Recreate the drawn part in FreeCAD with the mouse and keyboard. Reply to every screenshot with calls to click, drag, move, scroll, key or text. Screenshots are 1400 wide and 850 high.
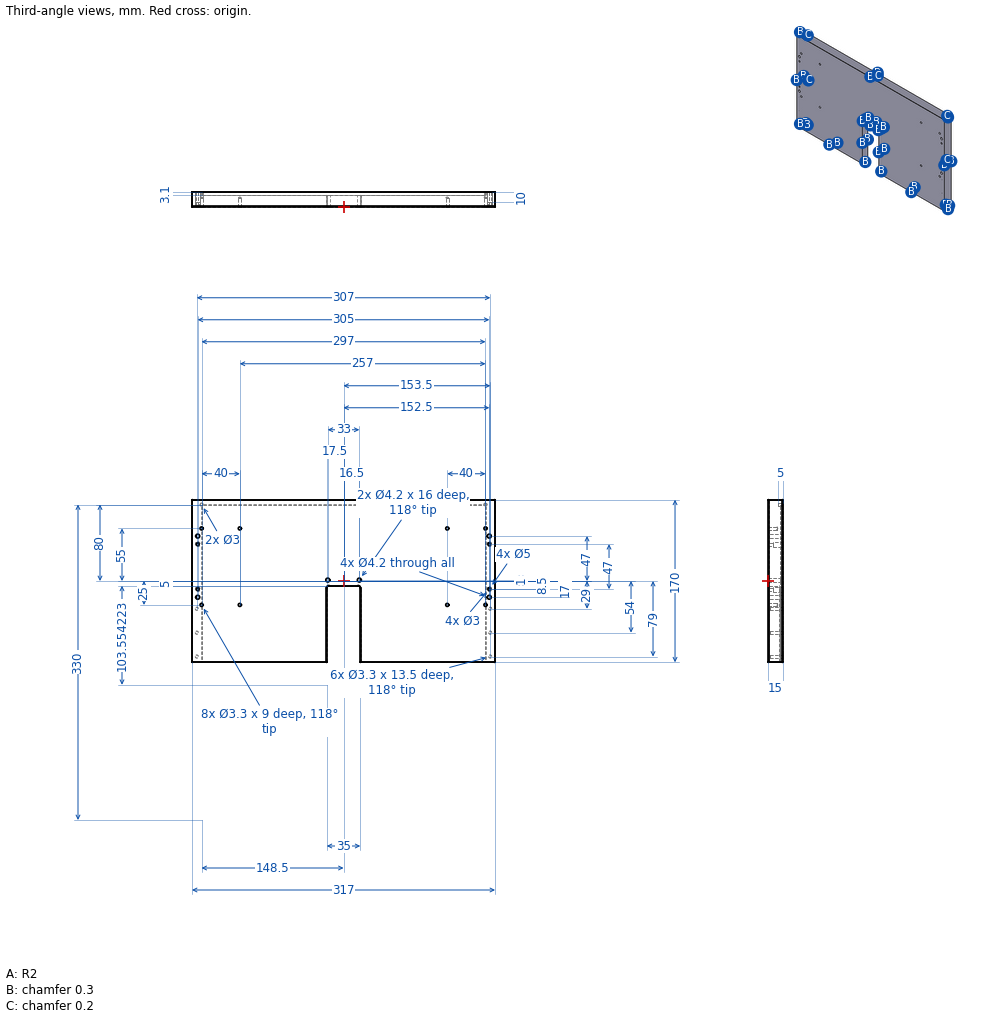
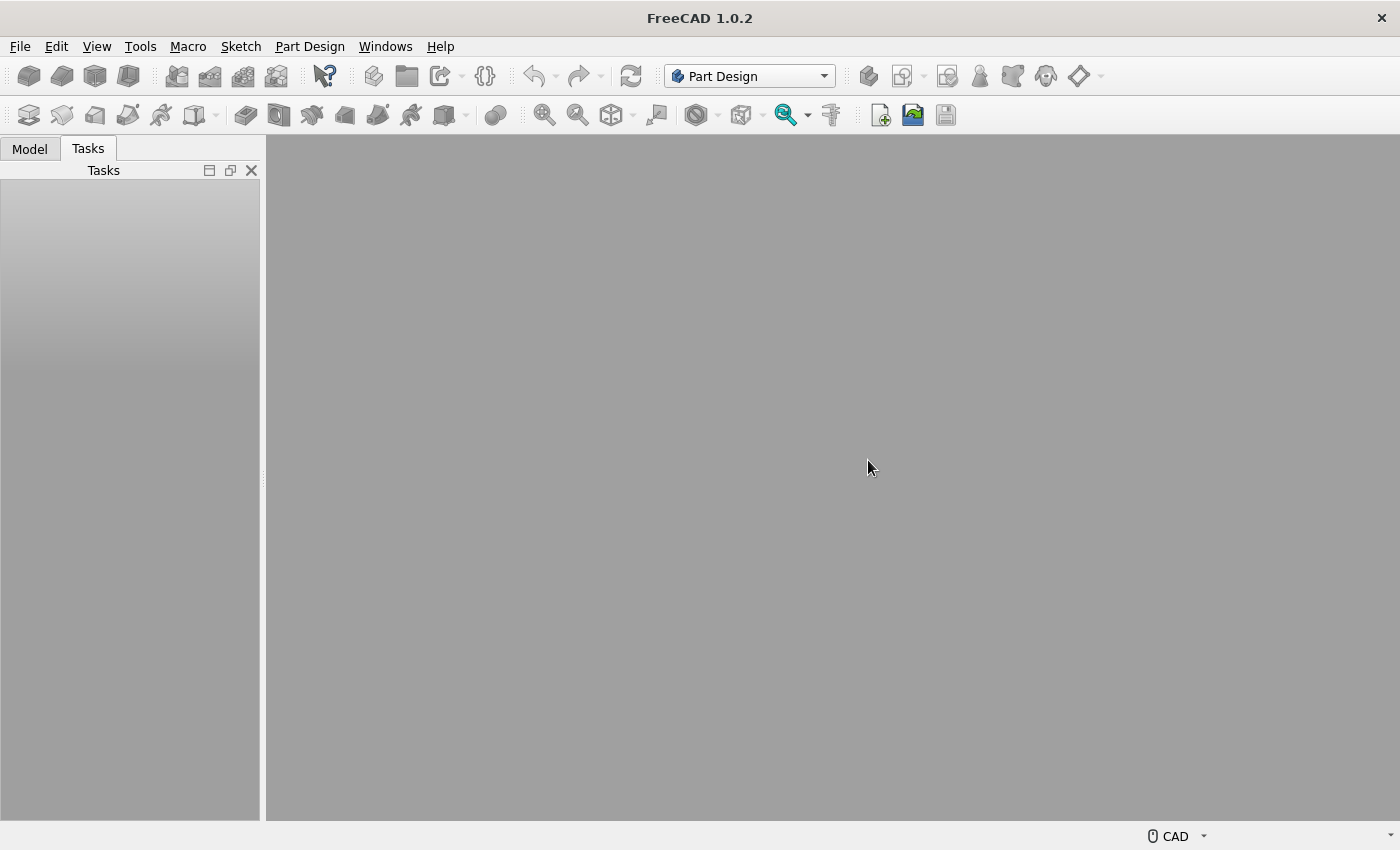
key(ctrl+n)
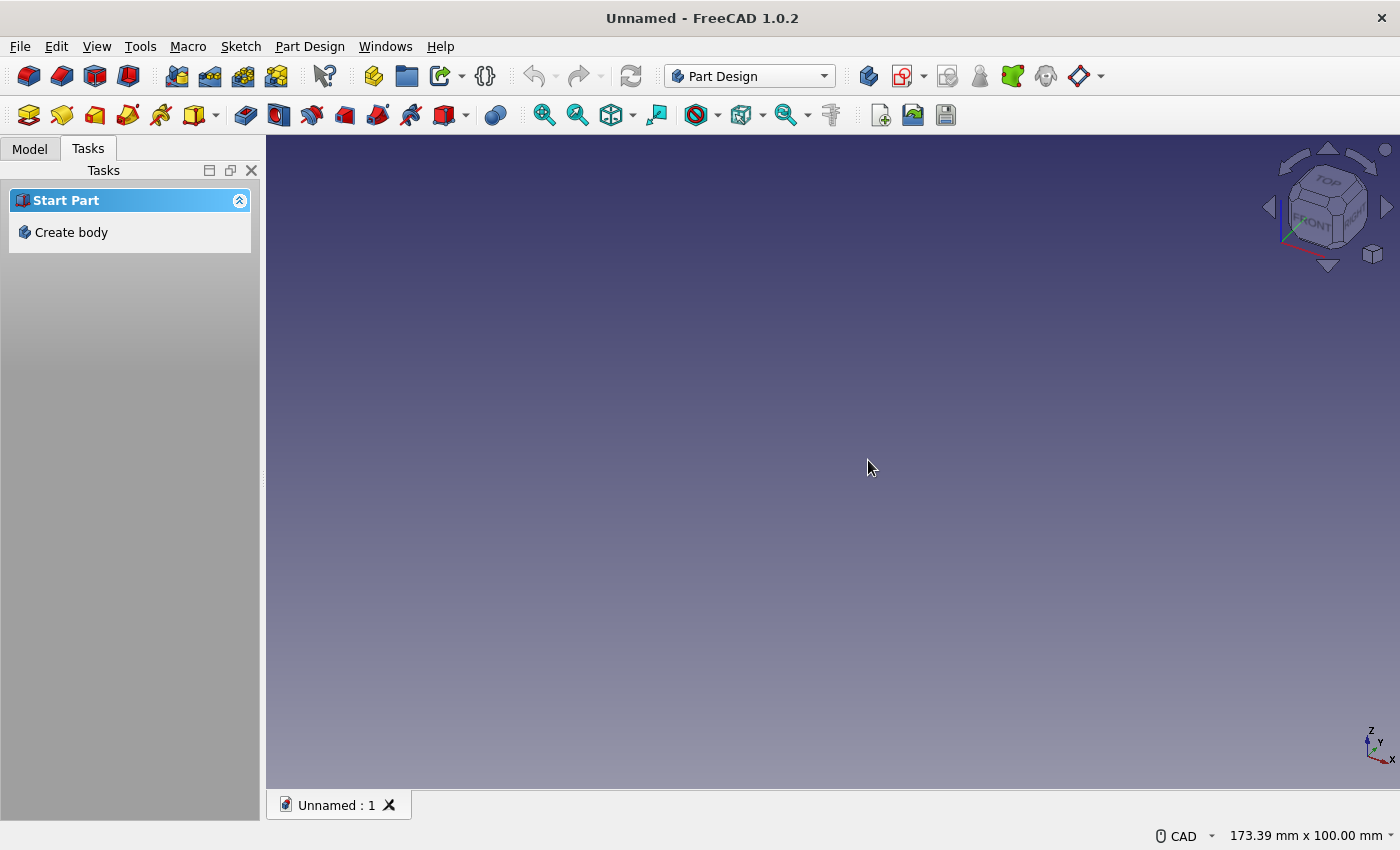
click(902, 76)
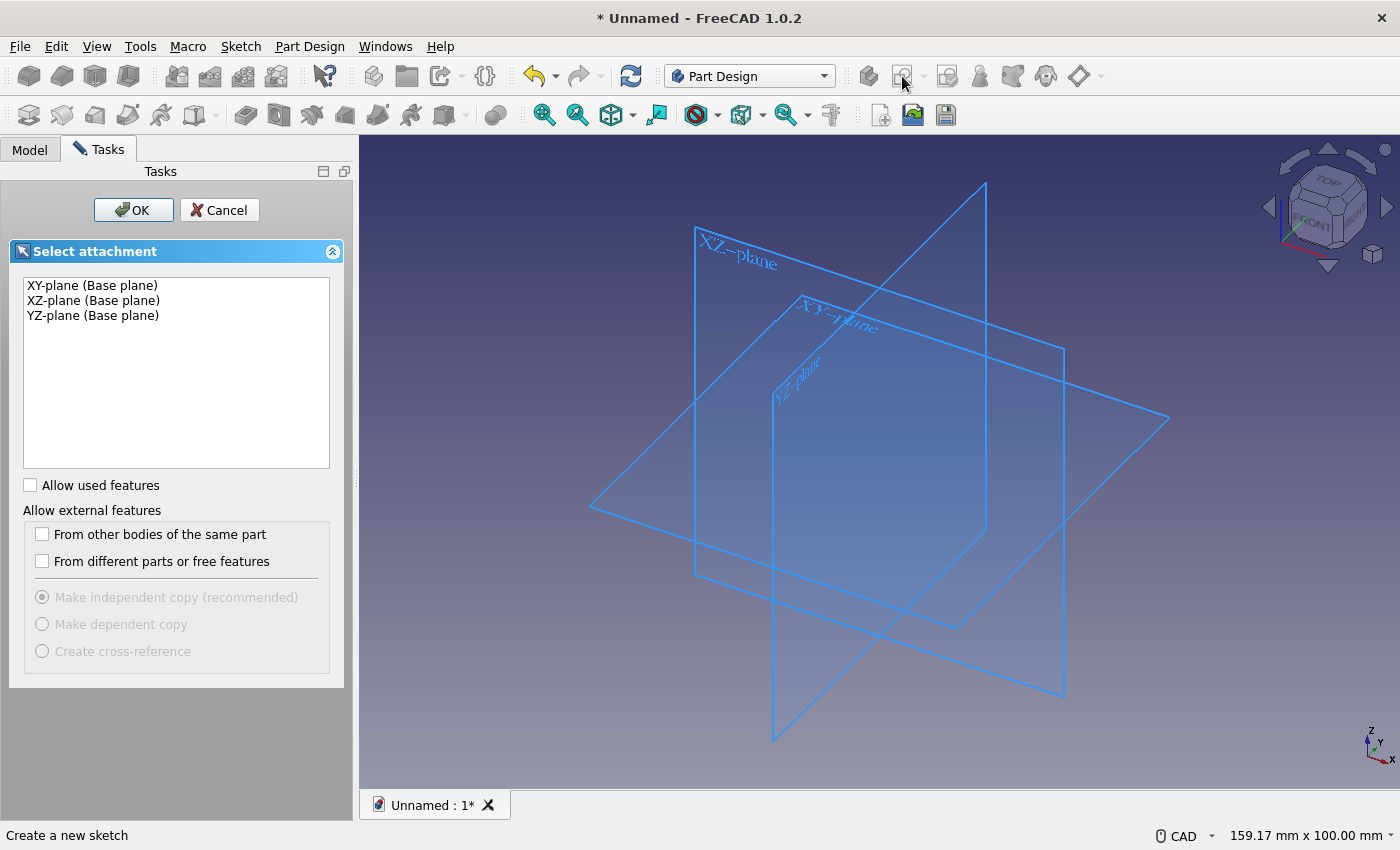
click(84, 300)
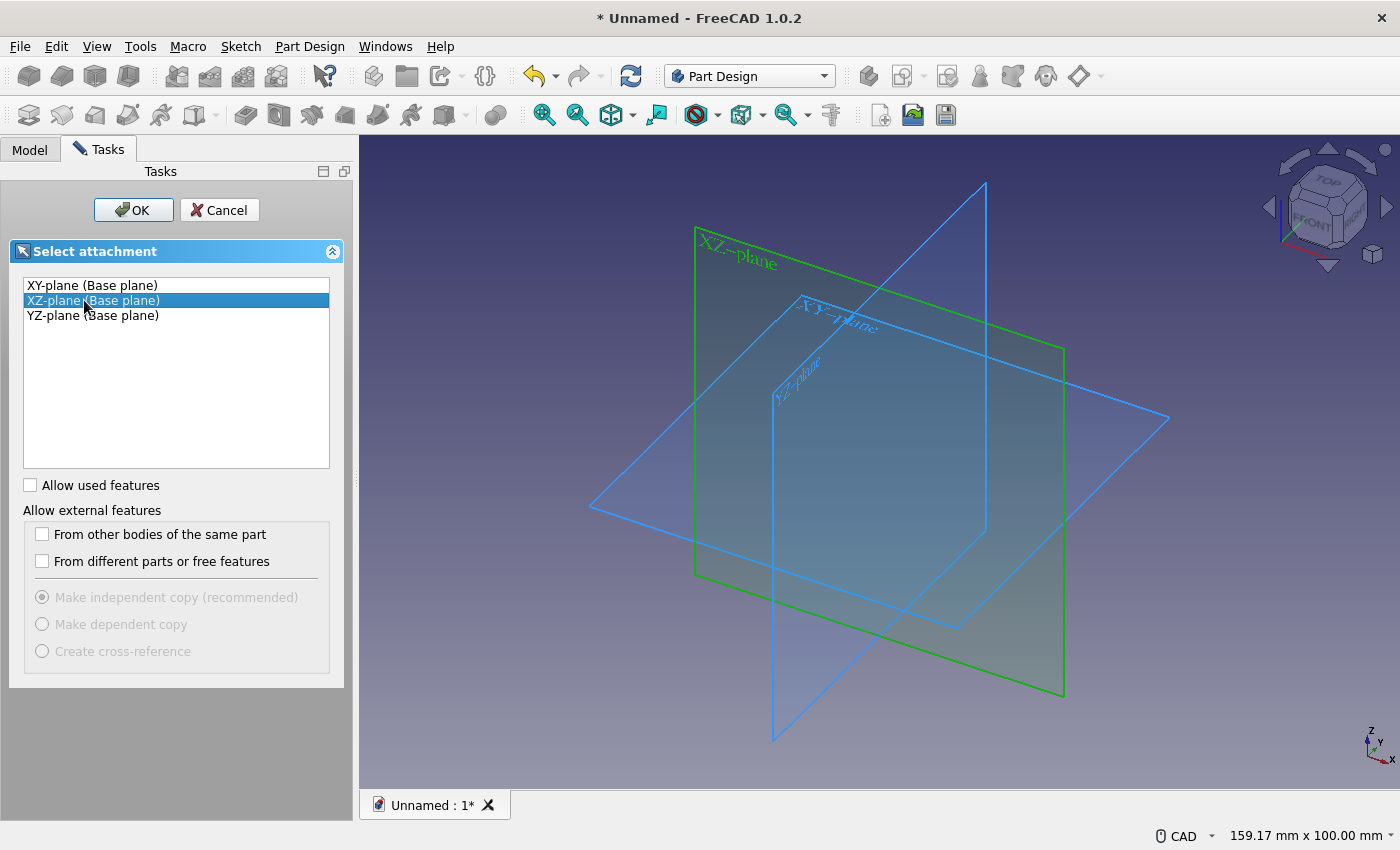
click(134, 210)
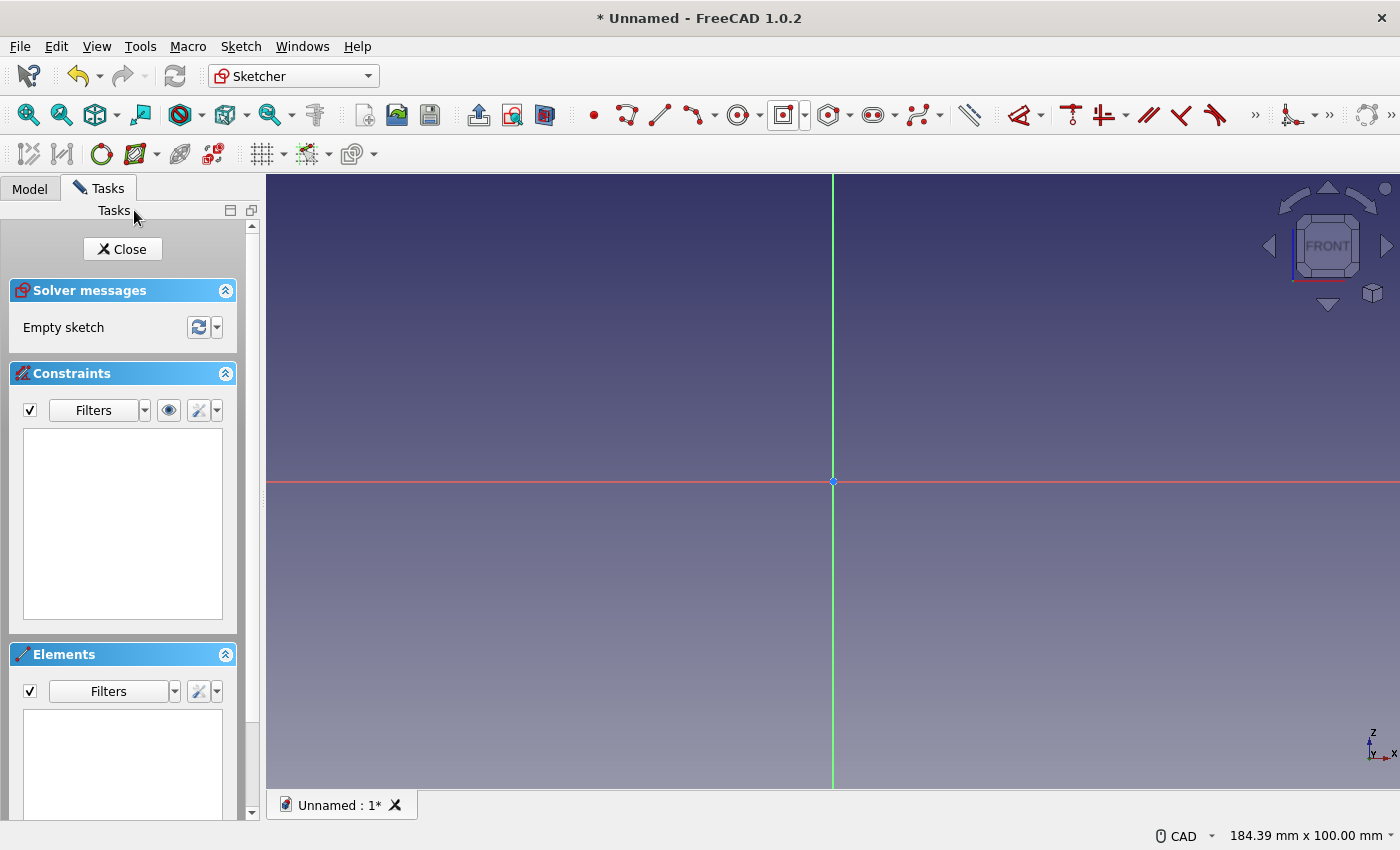
scroll(725, 482, down, 5)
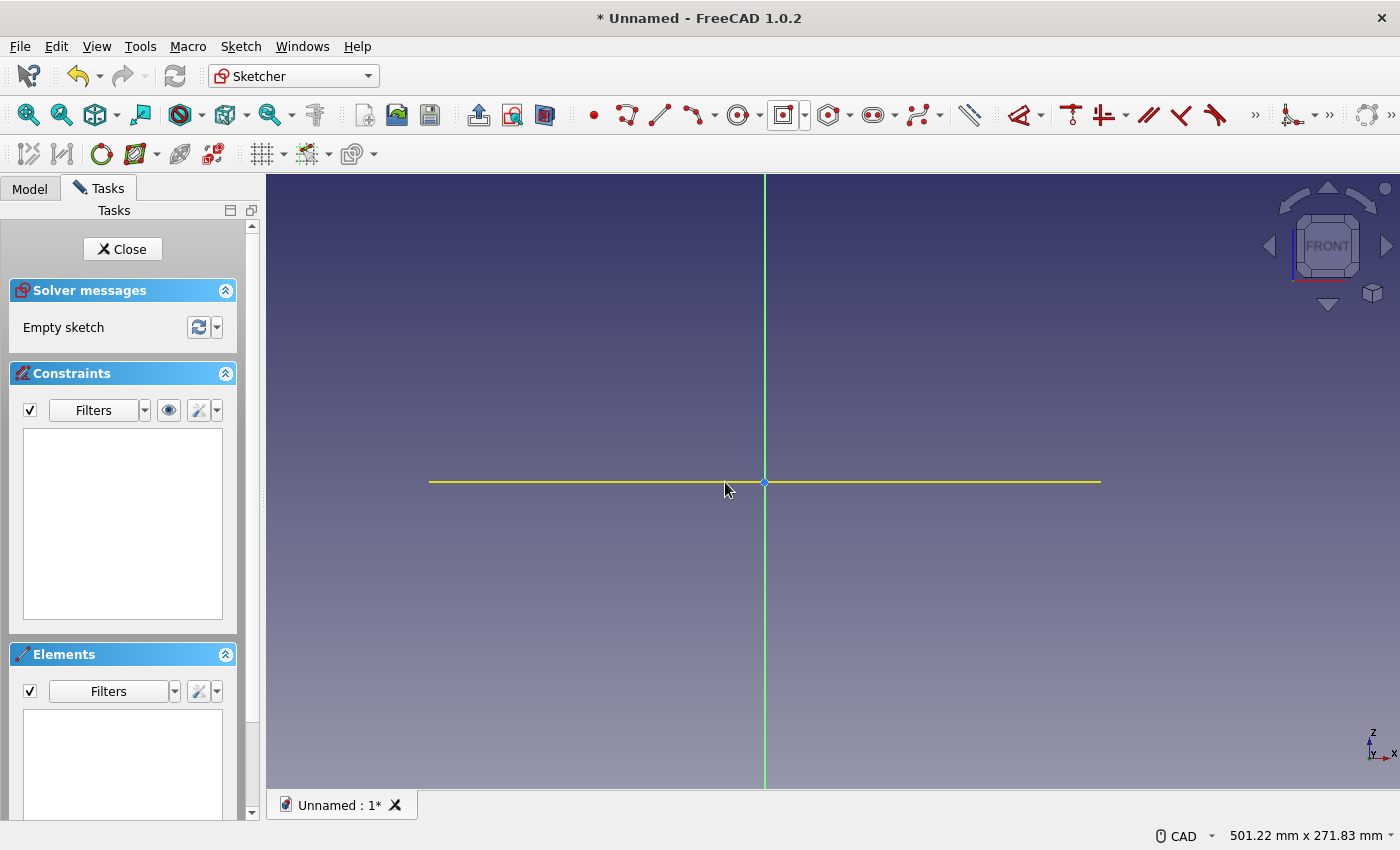
click(782, 116)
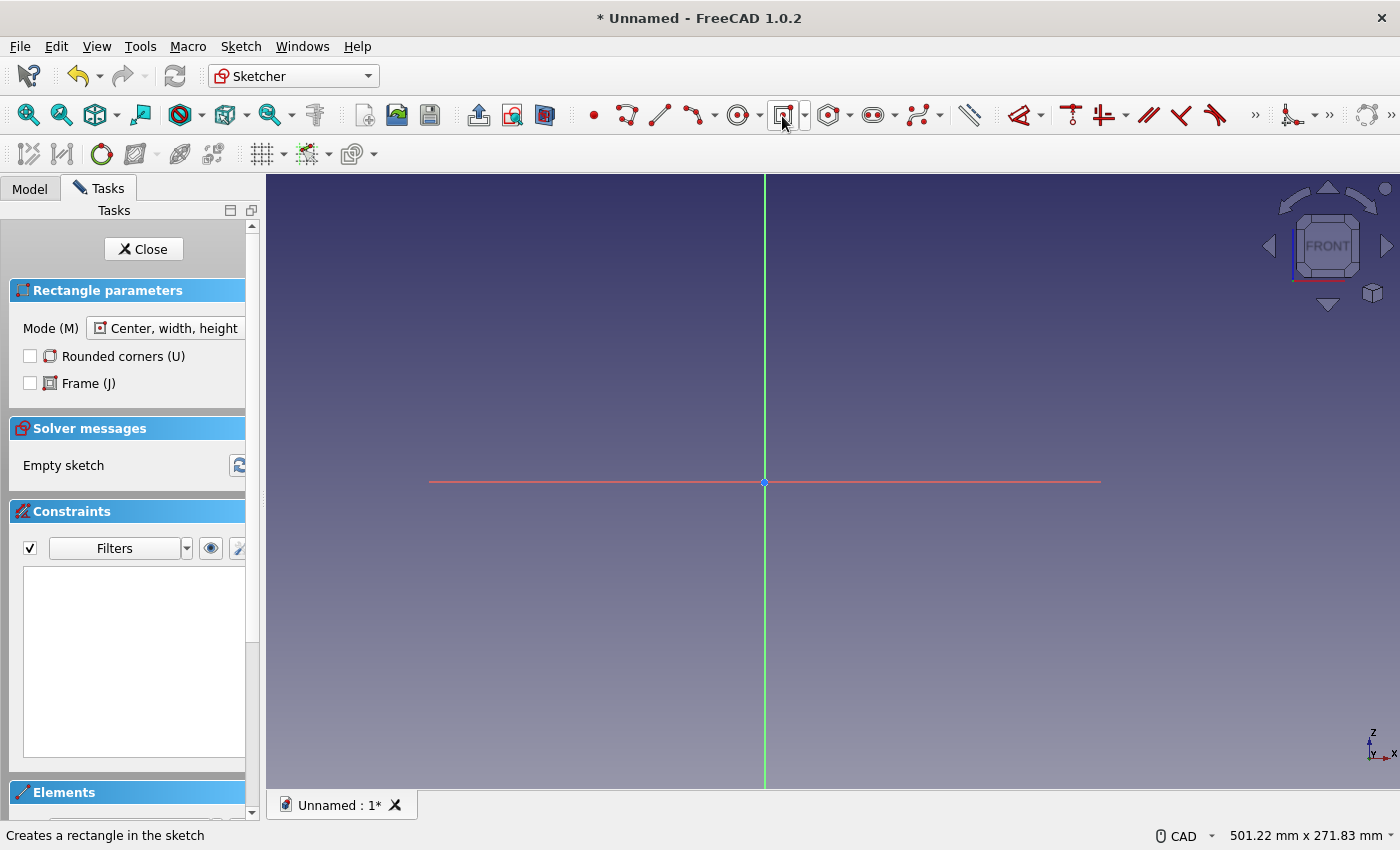
click(765, 482)
click(1124, 290)
key(Escape)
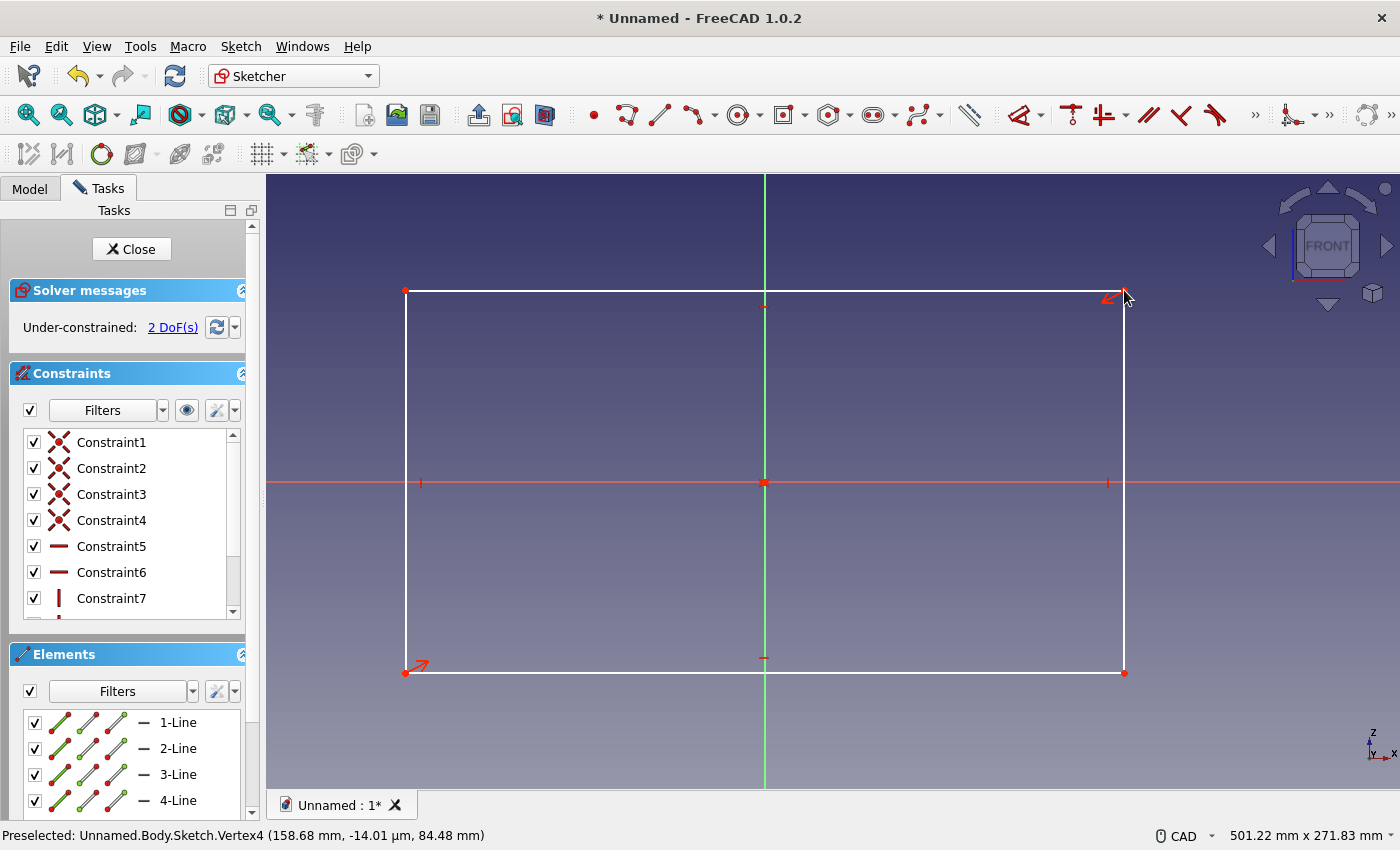
key(d)